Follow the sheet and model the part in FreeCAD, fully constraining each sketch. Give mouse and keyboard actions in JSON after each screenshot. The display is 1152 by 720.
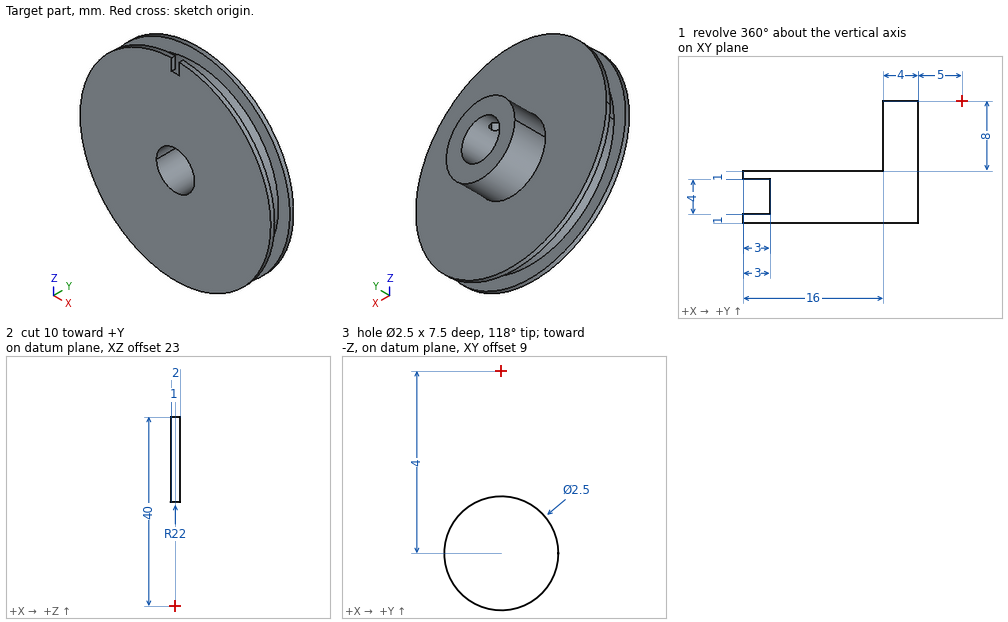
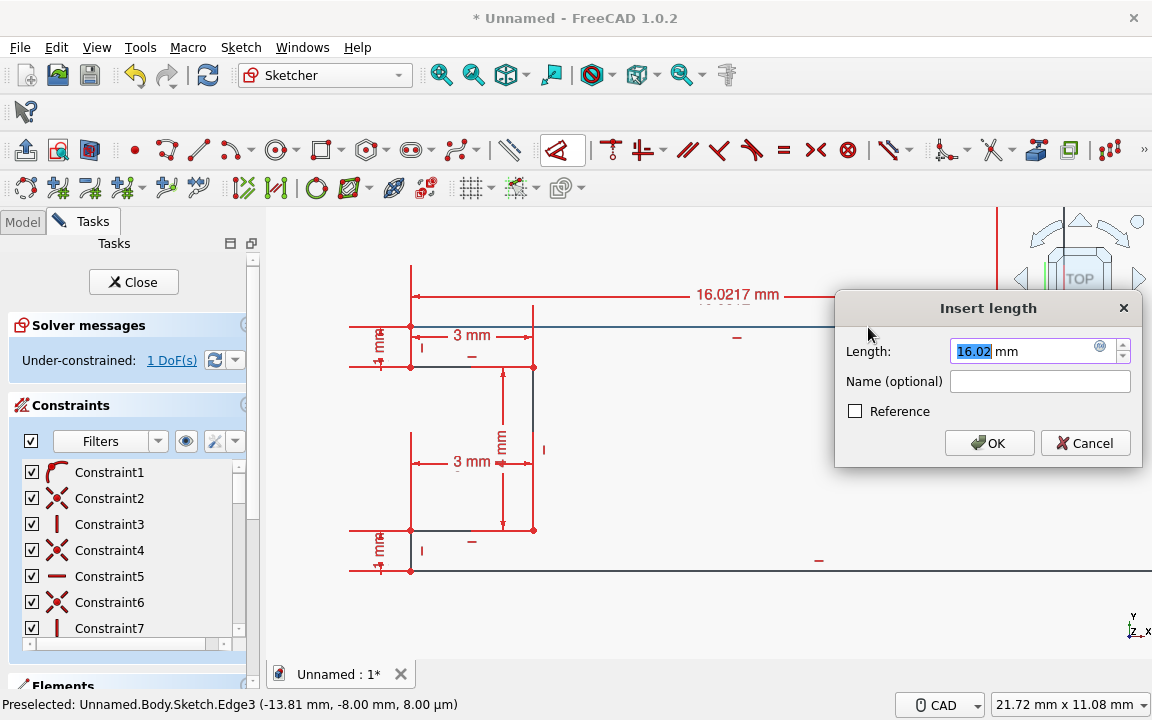
{"action": "type", "text": "16"}
{"action": "key", "text": "Return"}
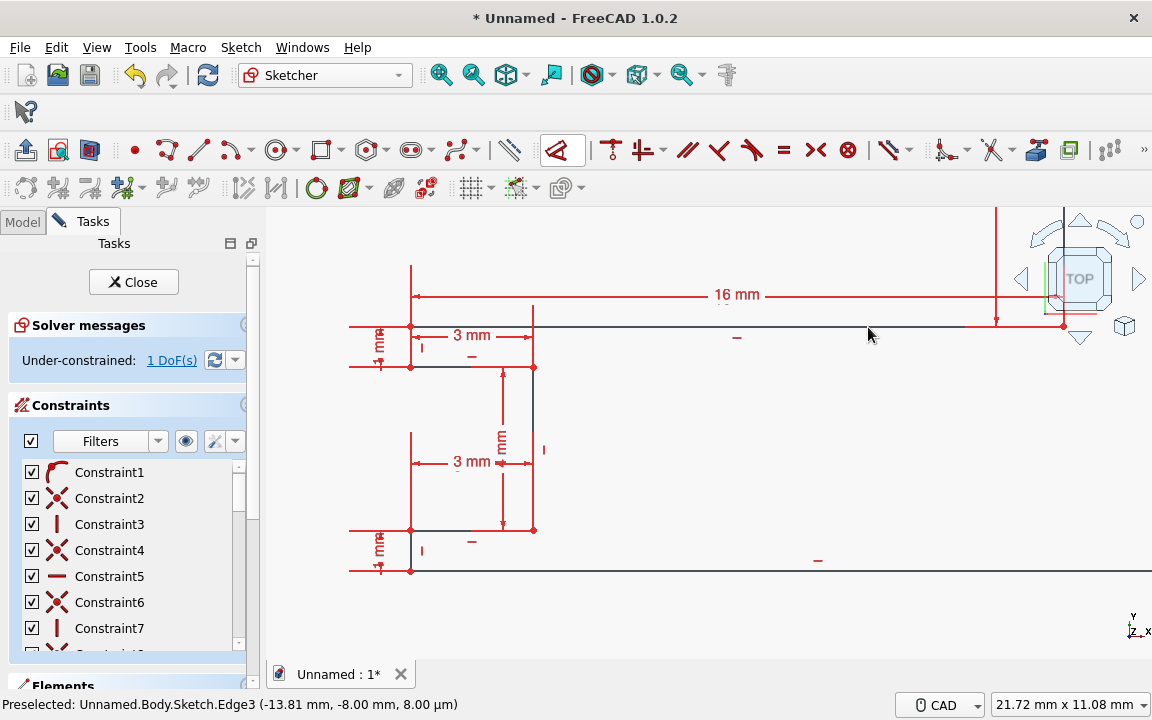
{"action": "scroll", "coordinate": [411, 553], "scroll_direction": "down", "scroll_amount": 4}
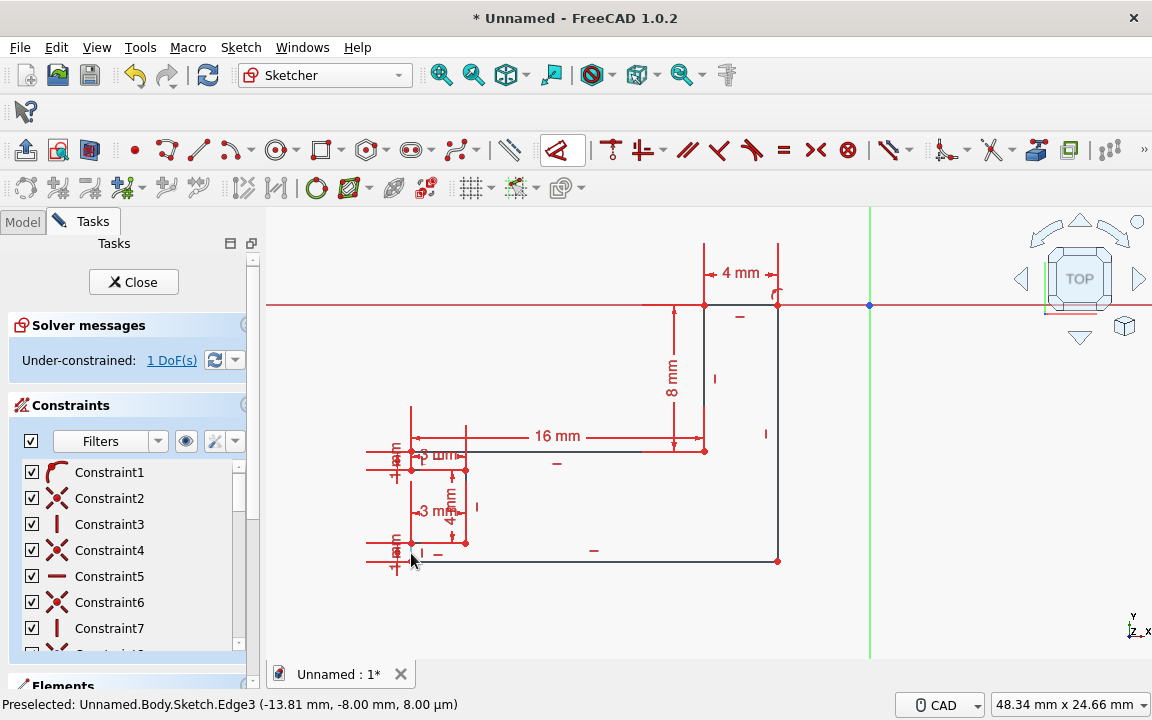
{"action": "left_click", "coordinate": [778, 305]}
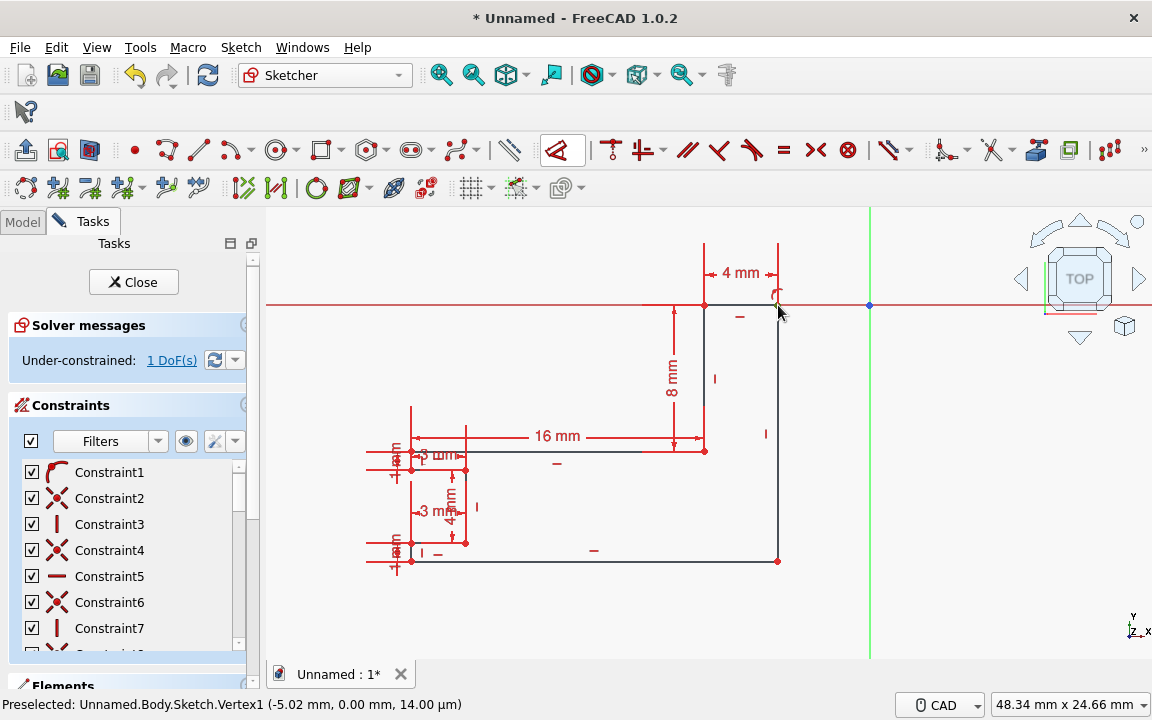
{"action": "left_click", "coordinate": [580, 150]}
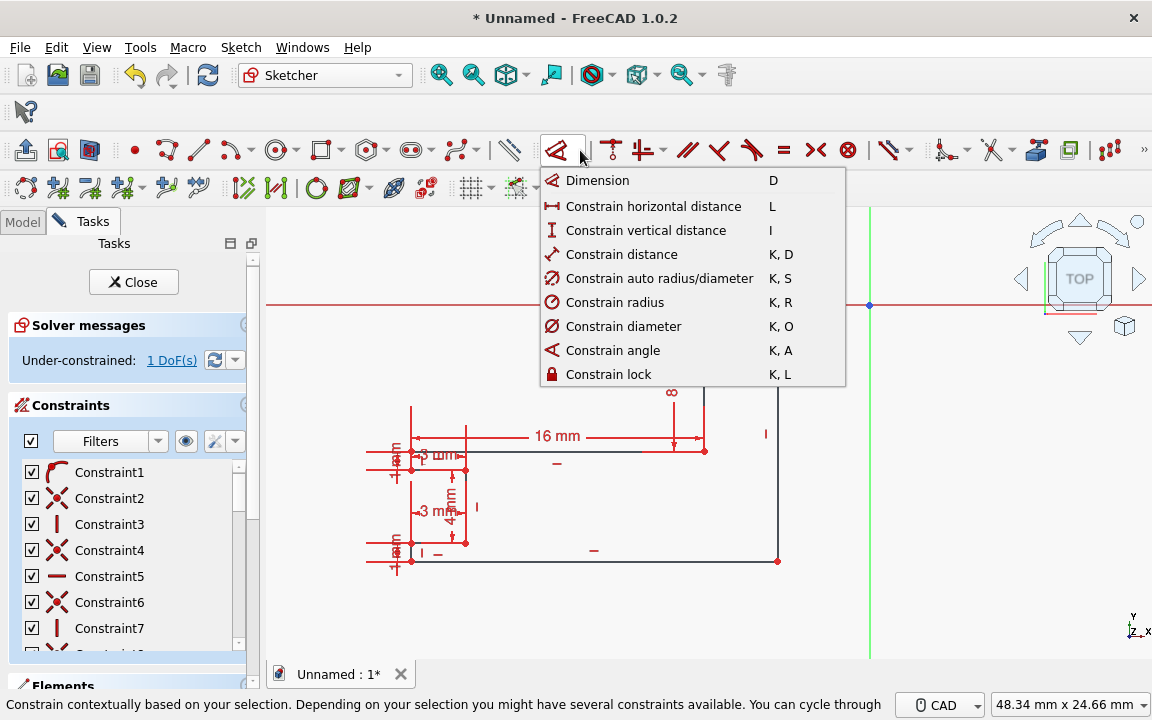
{"action": "left_click", "coordinate": [693, 206]}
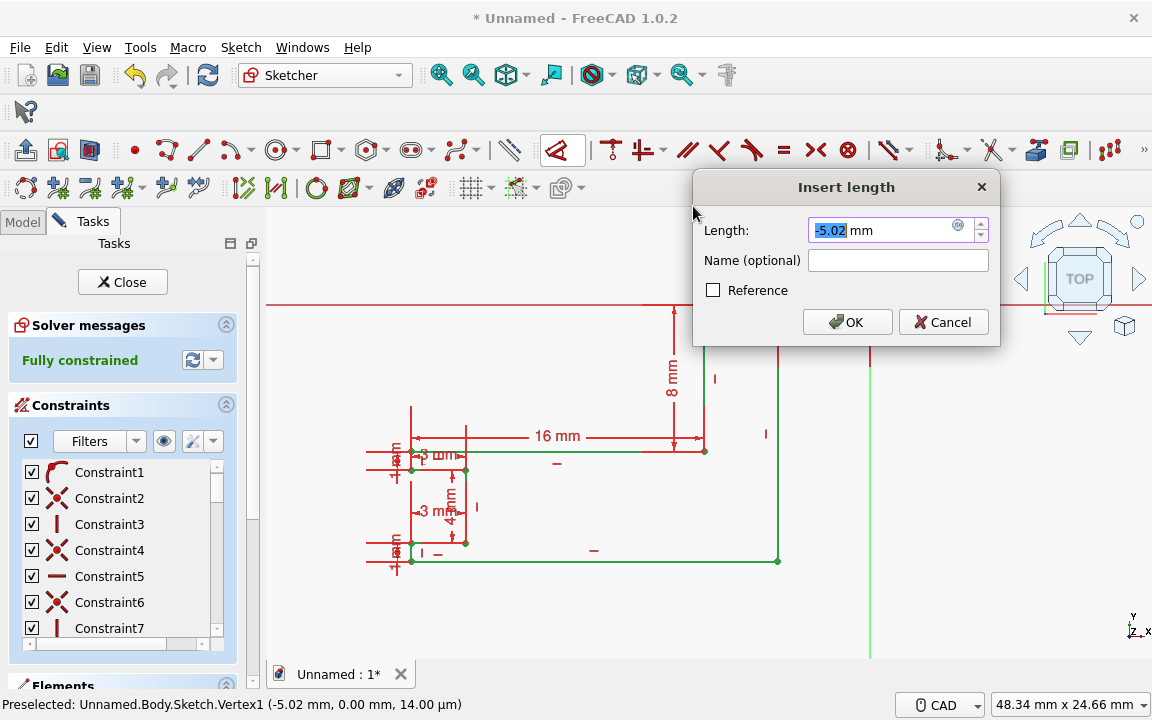
{"action": "type", "text": "-5"}
{"action": "key", "text": "Return"}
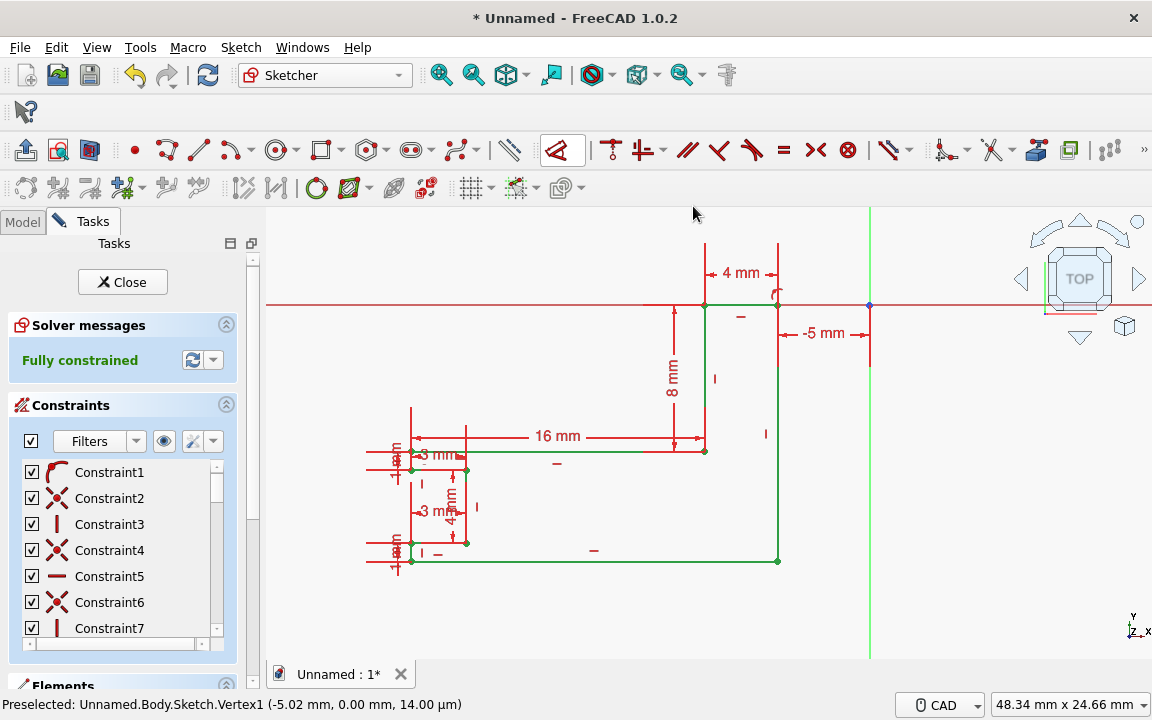
{"action": "left_click", "coordinate": [123, 282]}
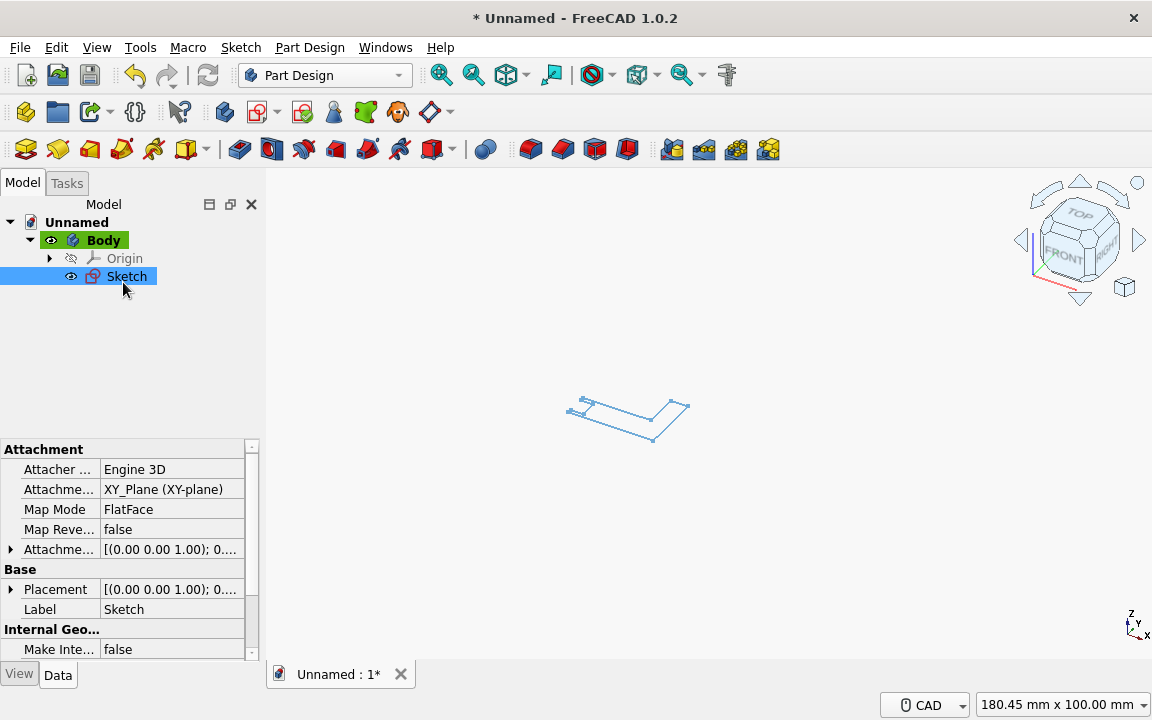
{"action": "left_click", "coordinate": [58, 150]}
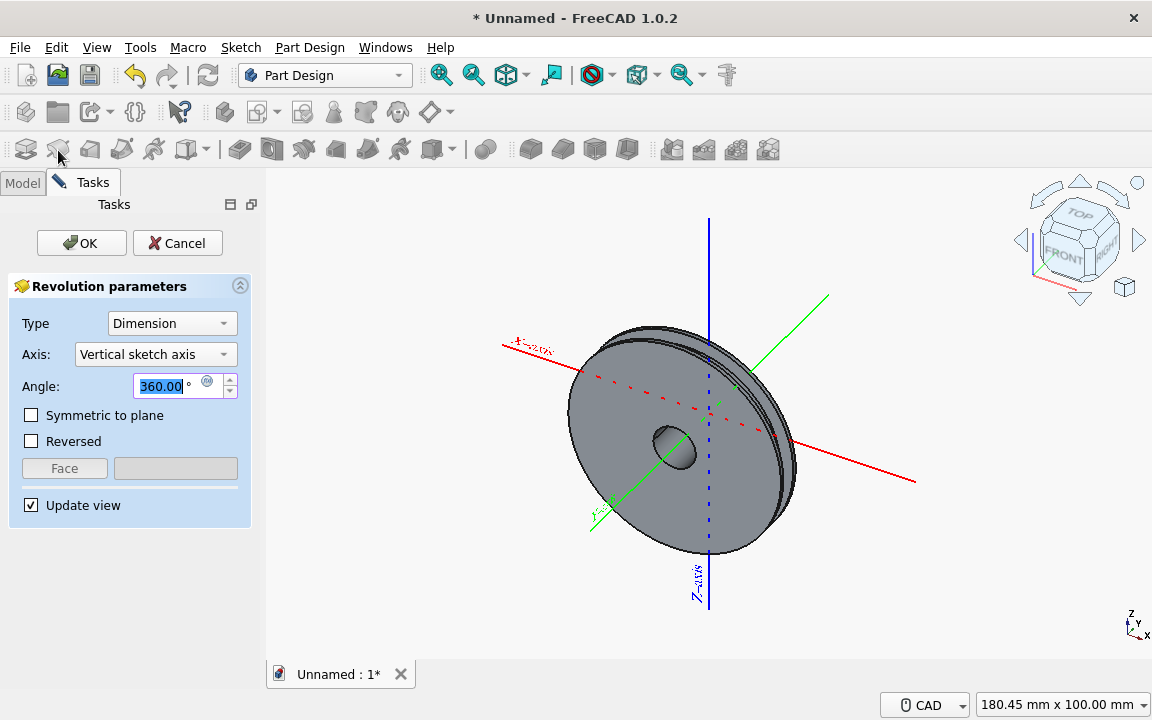
{"action": "left_click", "coordinate": [82, 243]}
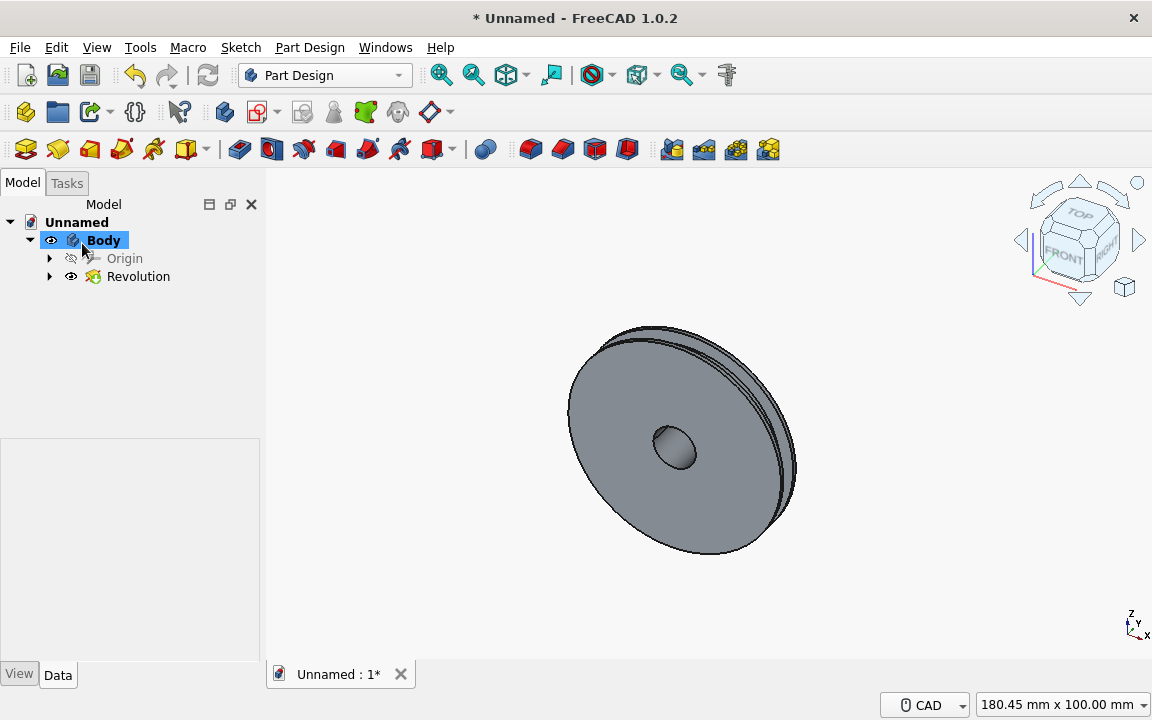
{"action": "left_click", "coordinate": [50, 258]}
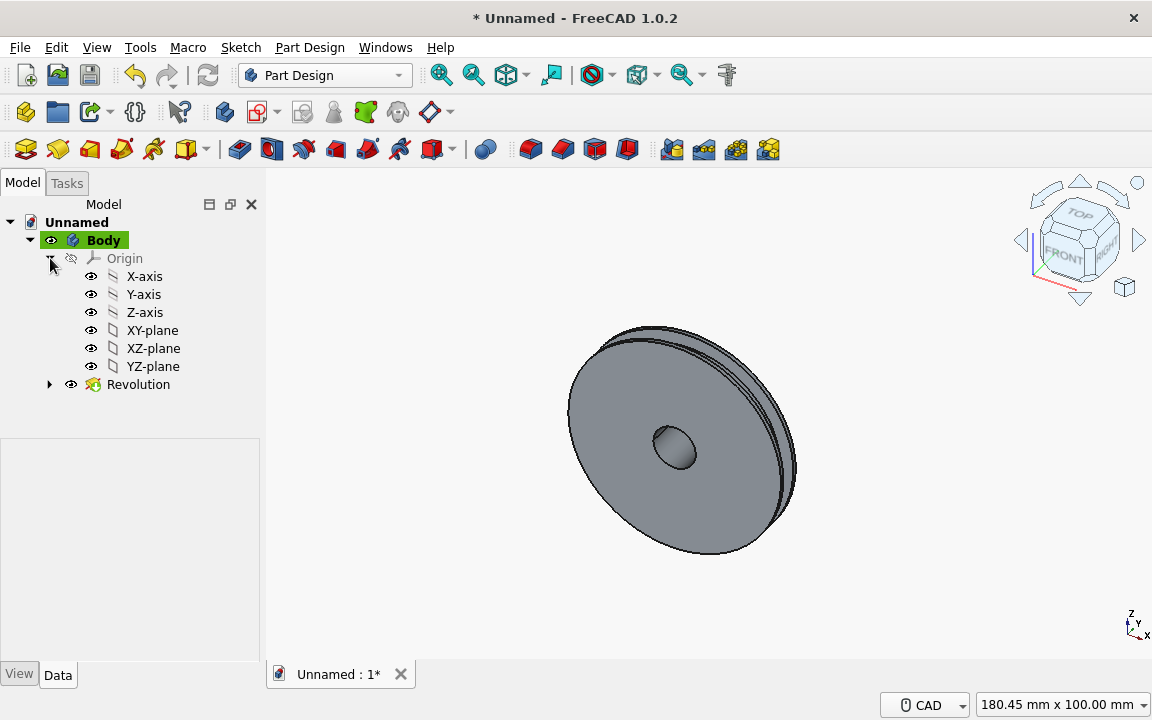
{"action": "left_click", "coordinate": [136, 348]}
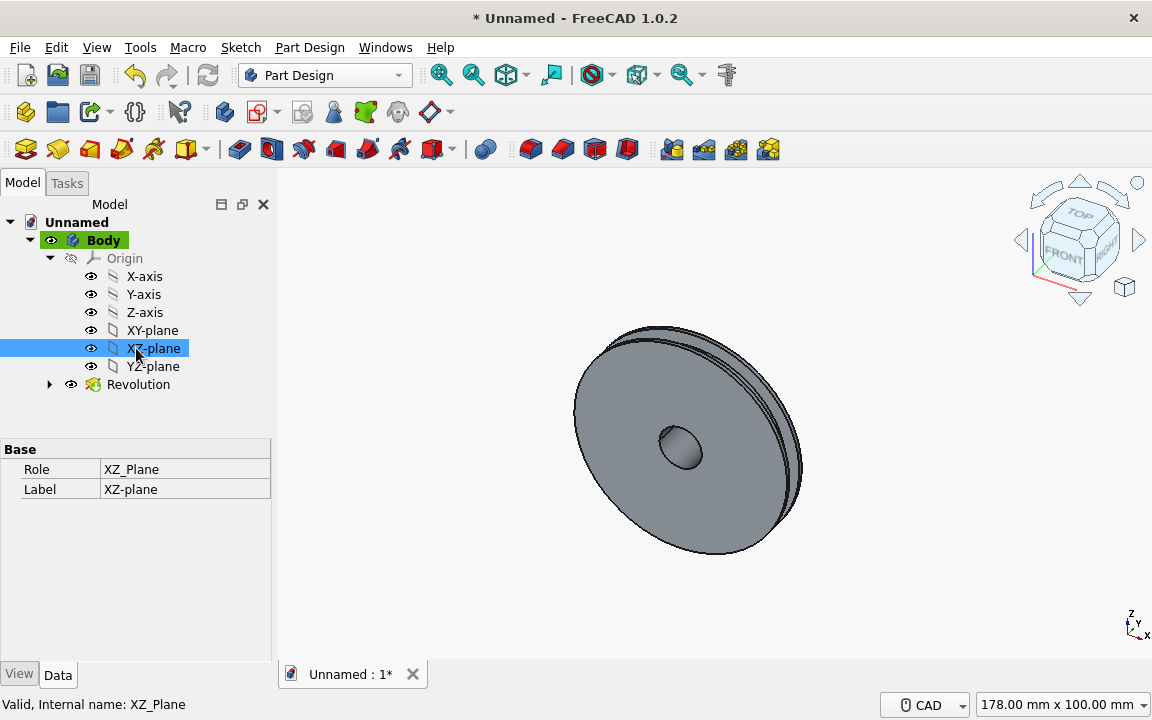
{"action": "left_click", "coordinate": [430, 112]}